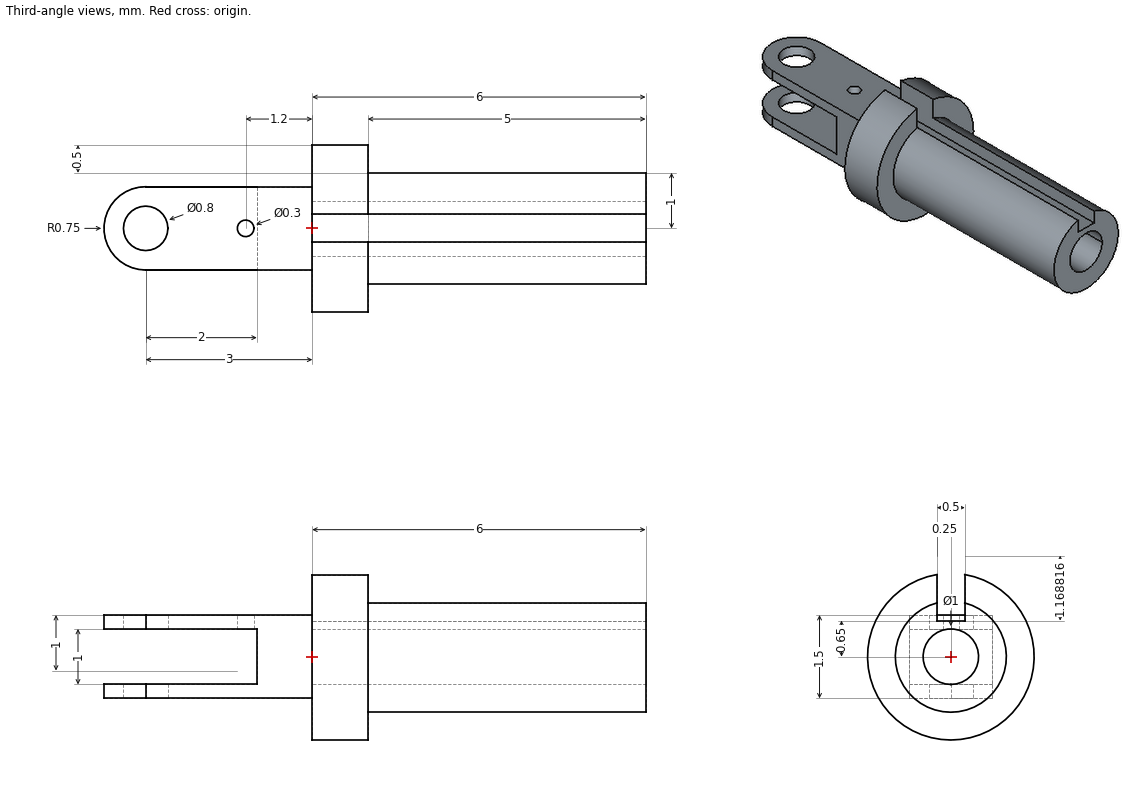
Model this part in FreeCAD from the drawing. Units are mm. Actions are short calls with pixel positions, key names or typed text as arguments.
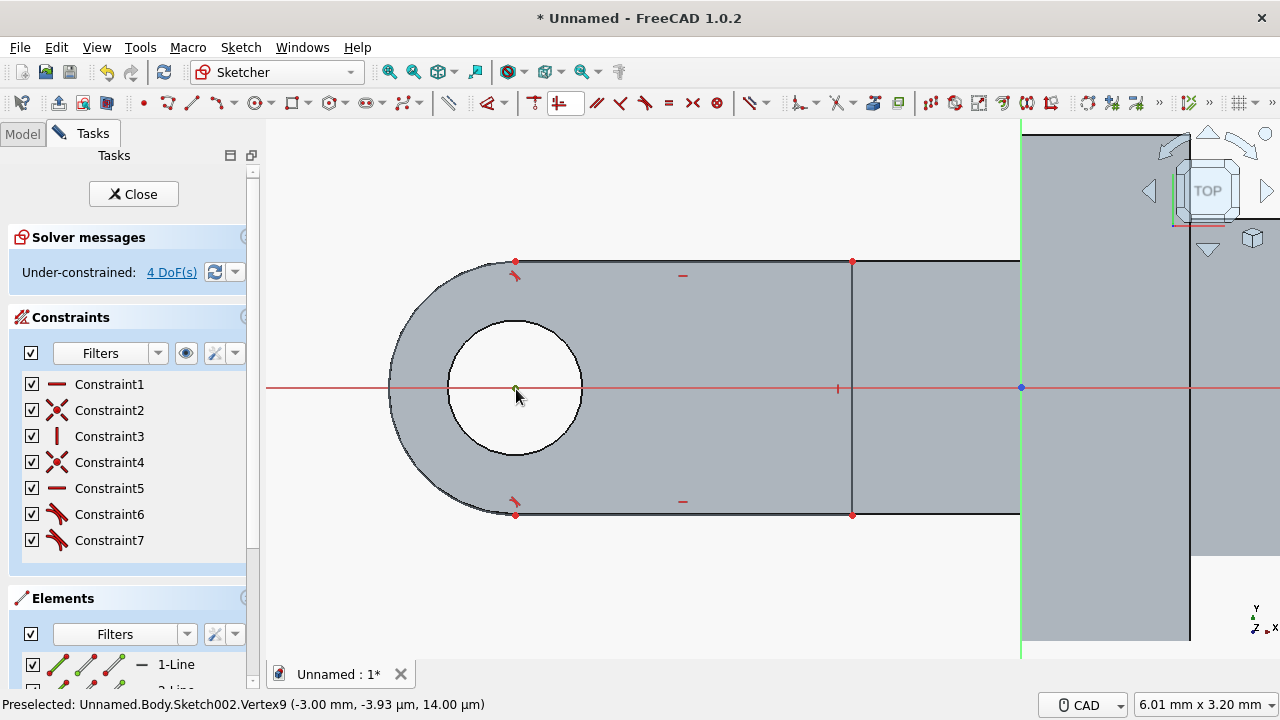
click(353, 388)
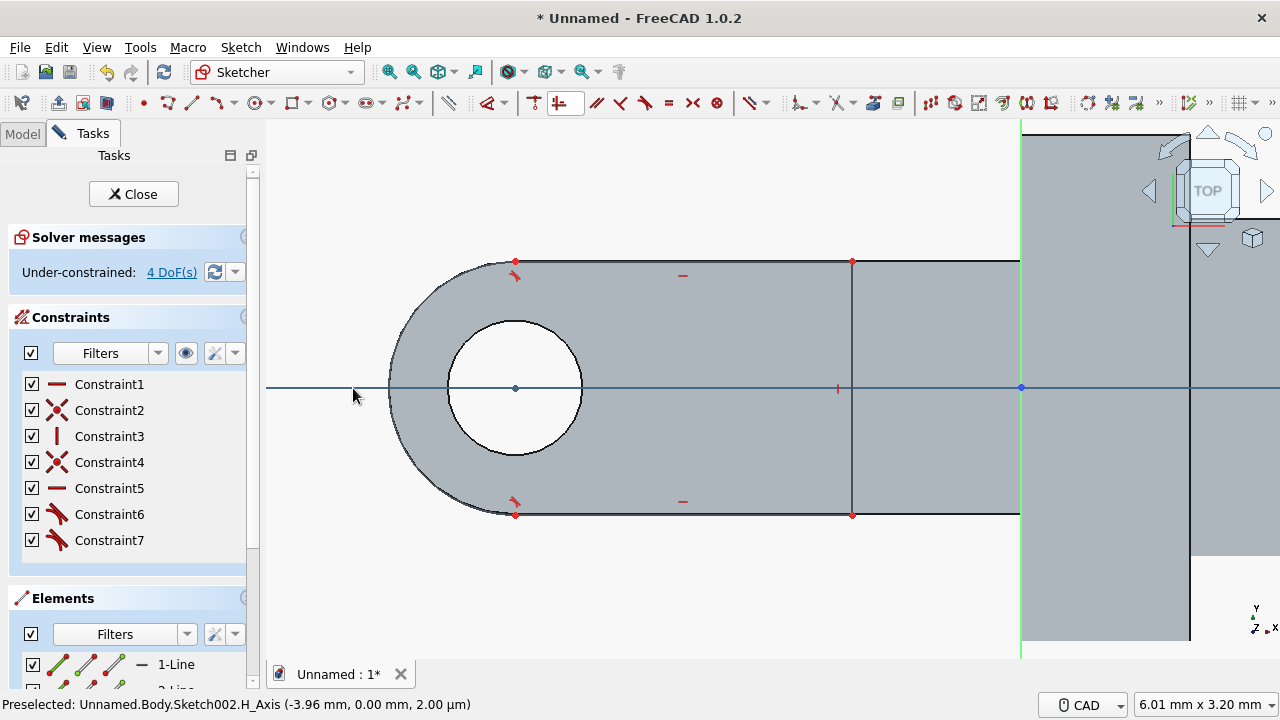
click(534, 104)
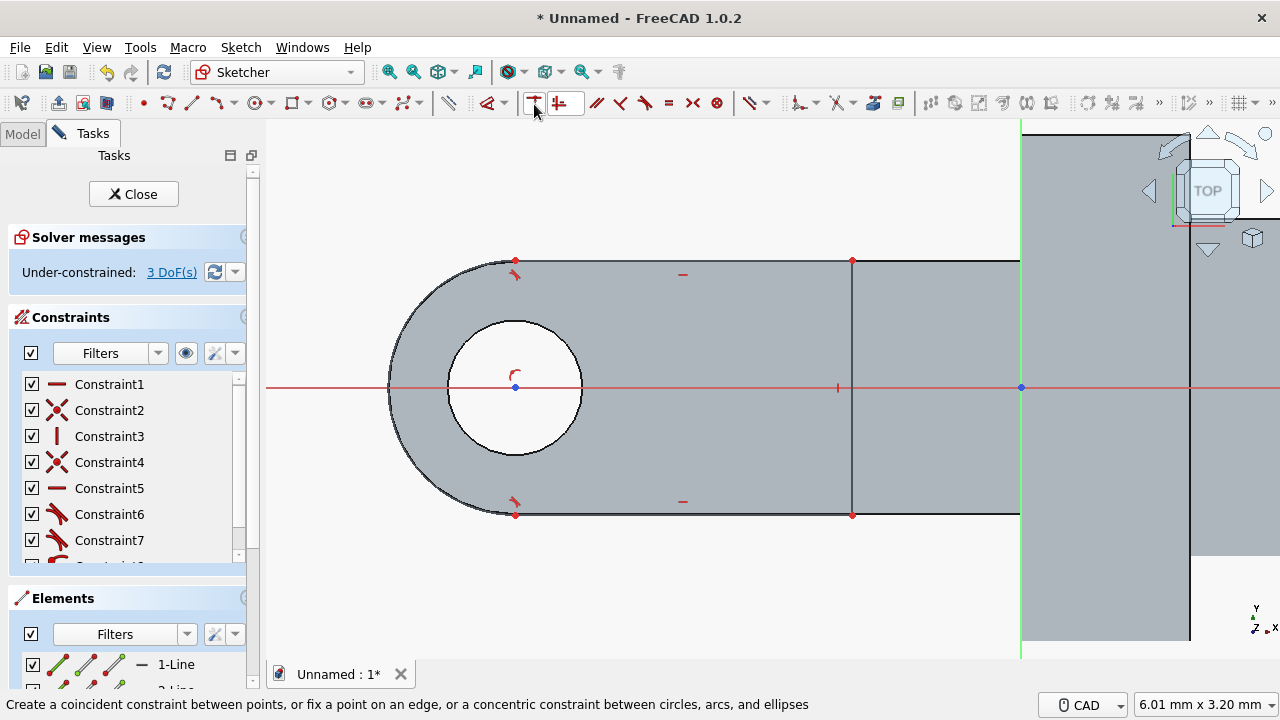
click(488, 104)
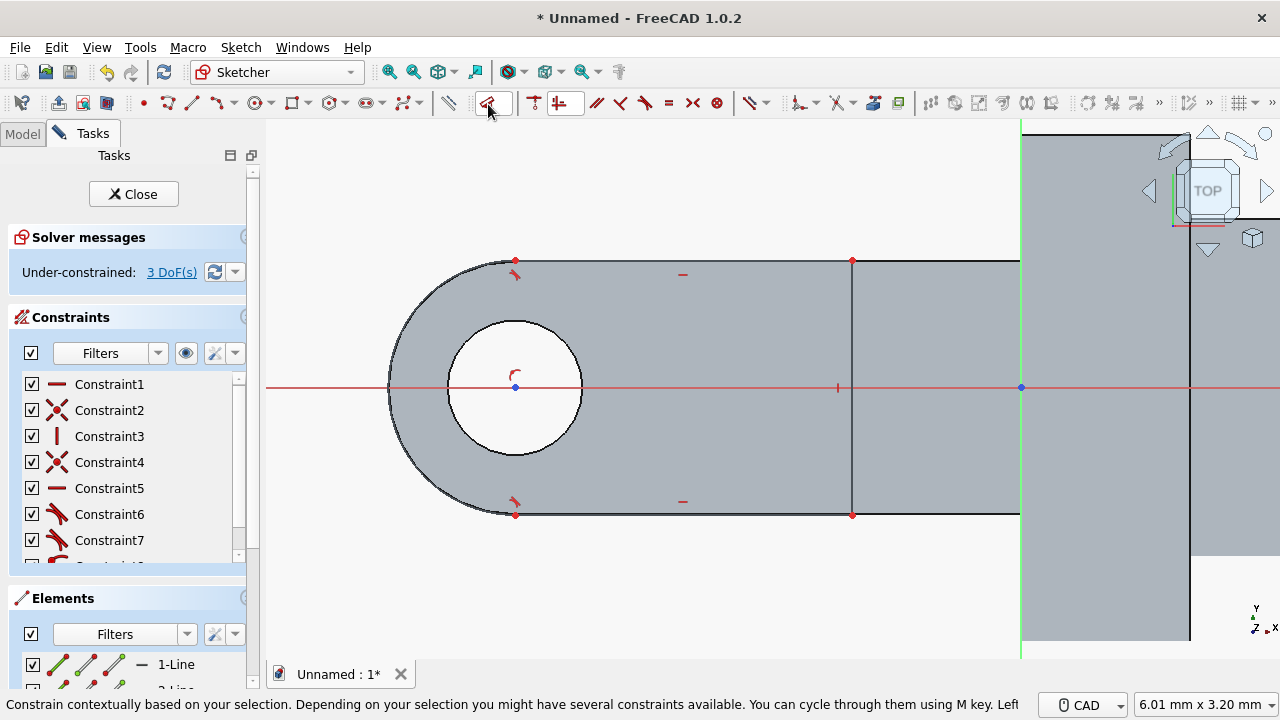
click(413, 313)
click(387, 294)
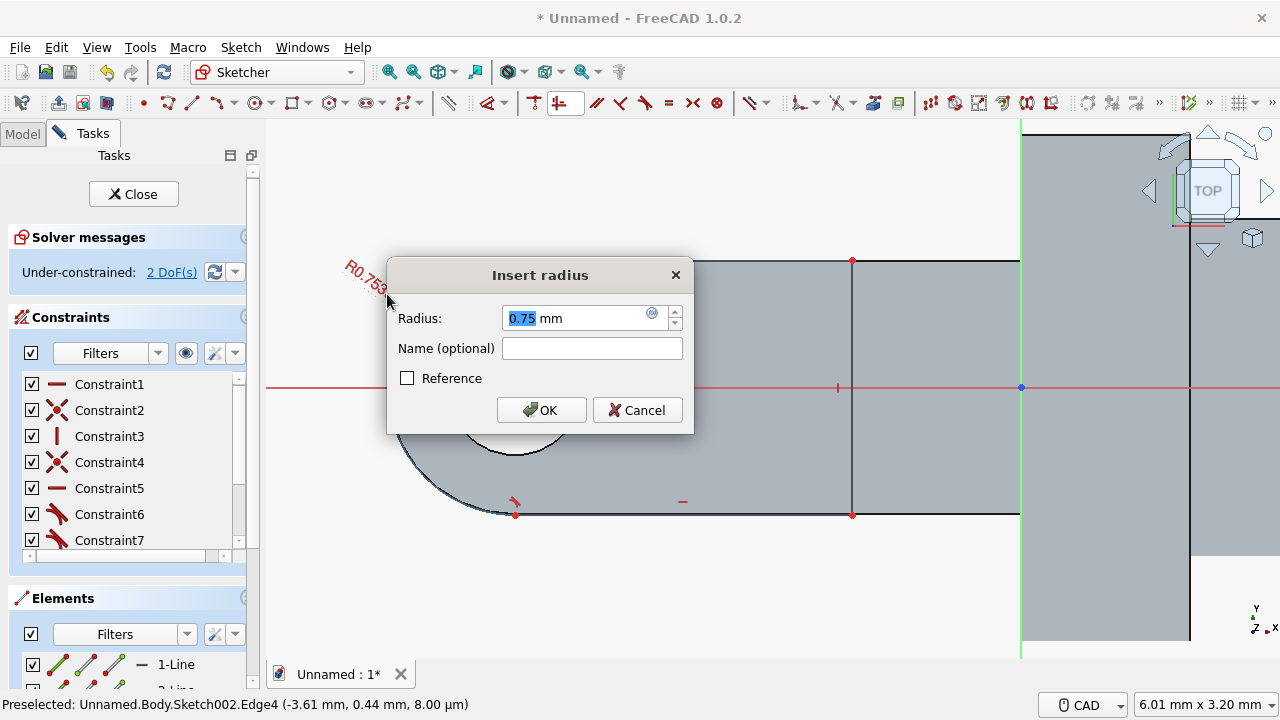
text(0.75)
key(Return)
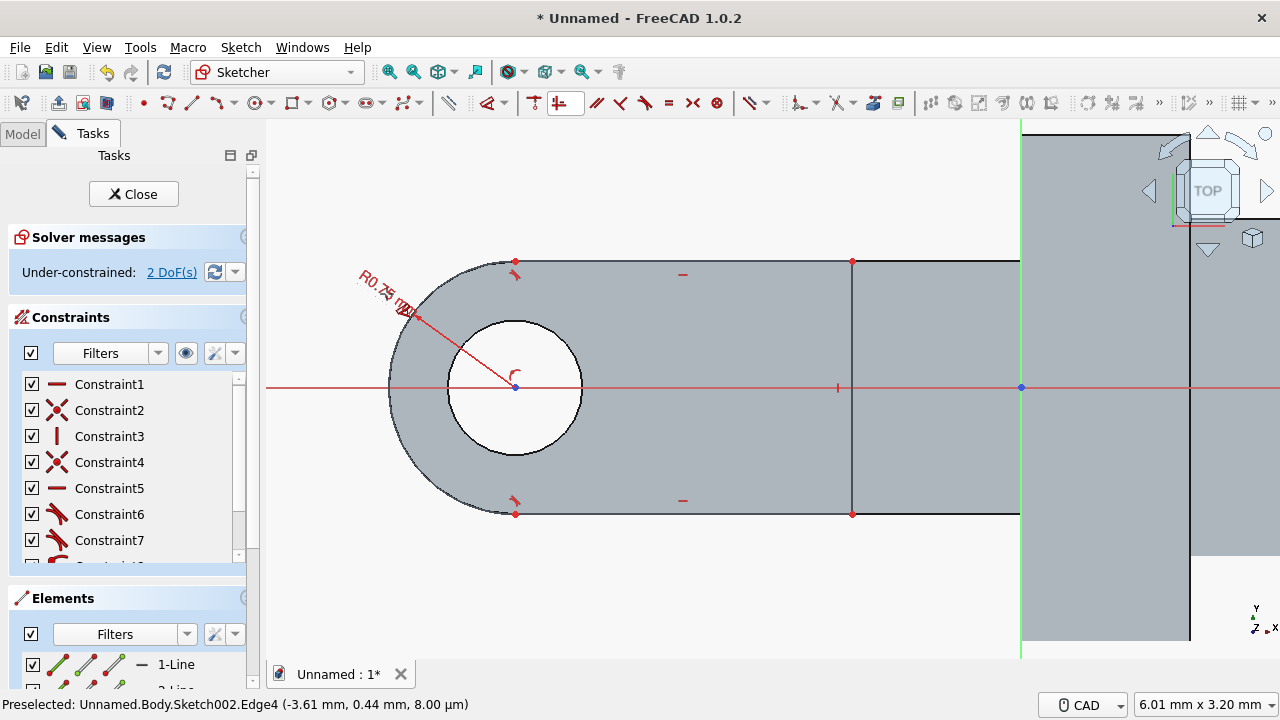
click(616, 514)
click(684, 548)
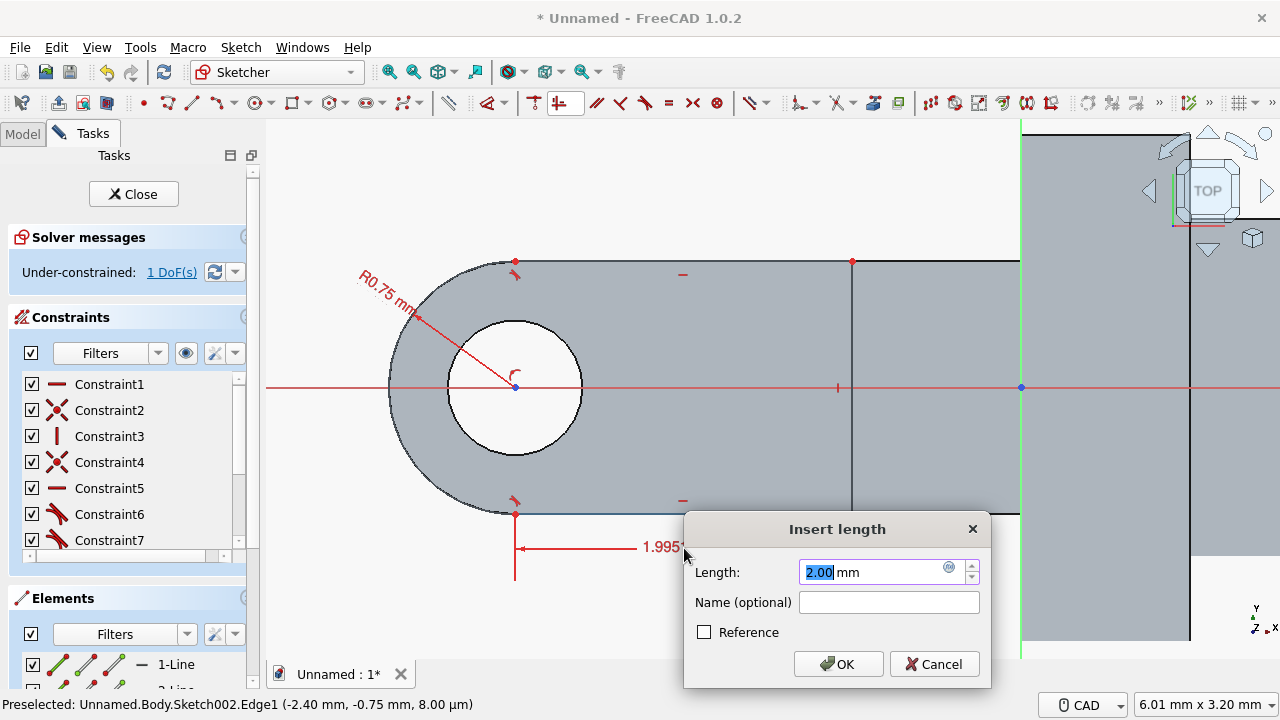
text(2)
key(Return)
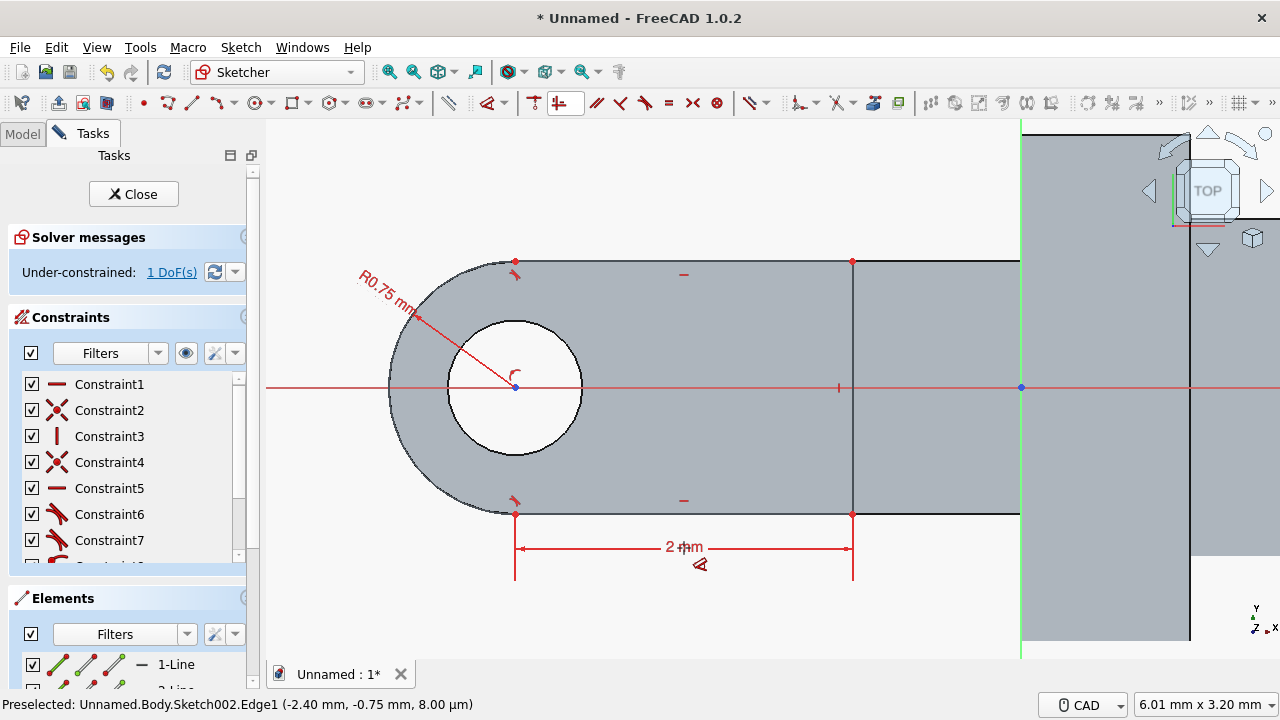
click(516, 514)
click(768, 548)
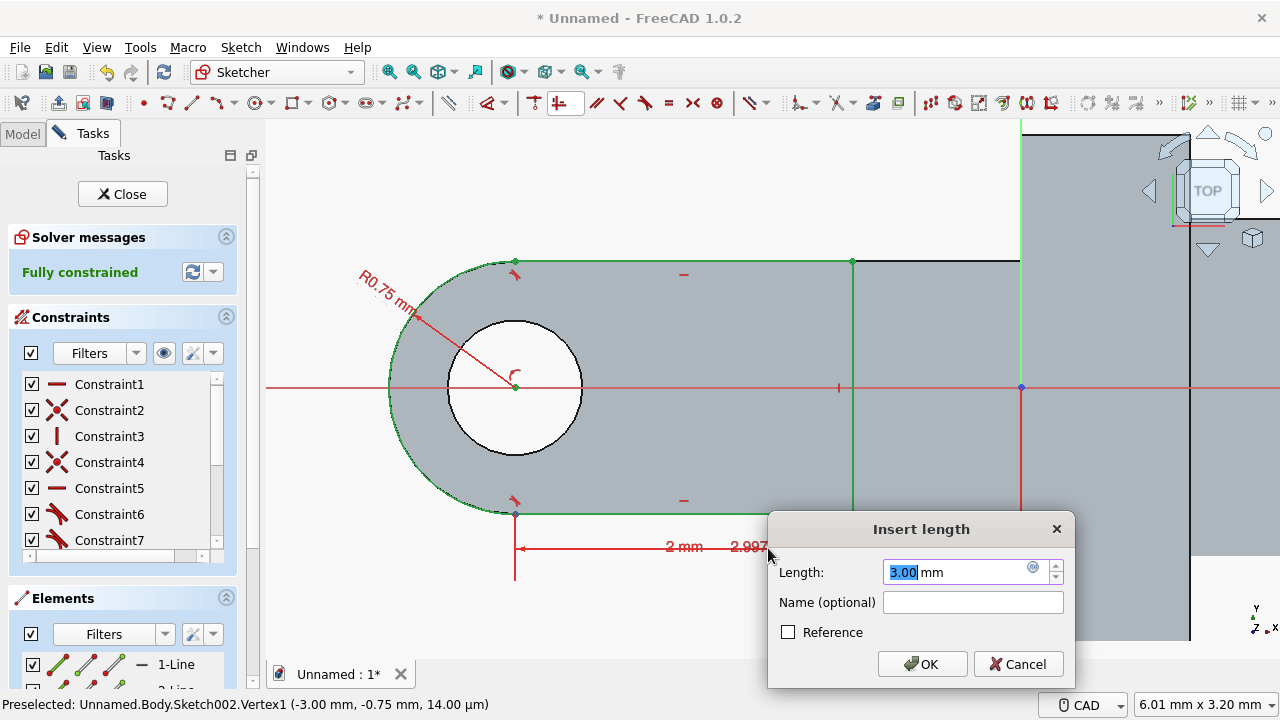
text(3)
key(Return)
key(Escape)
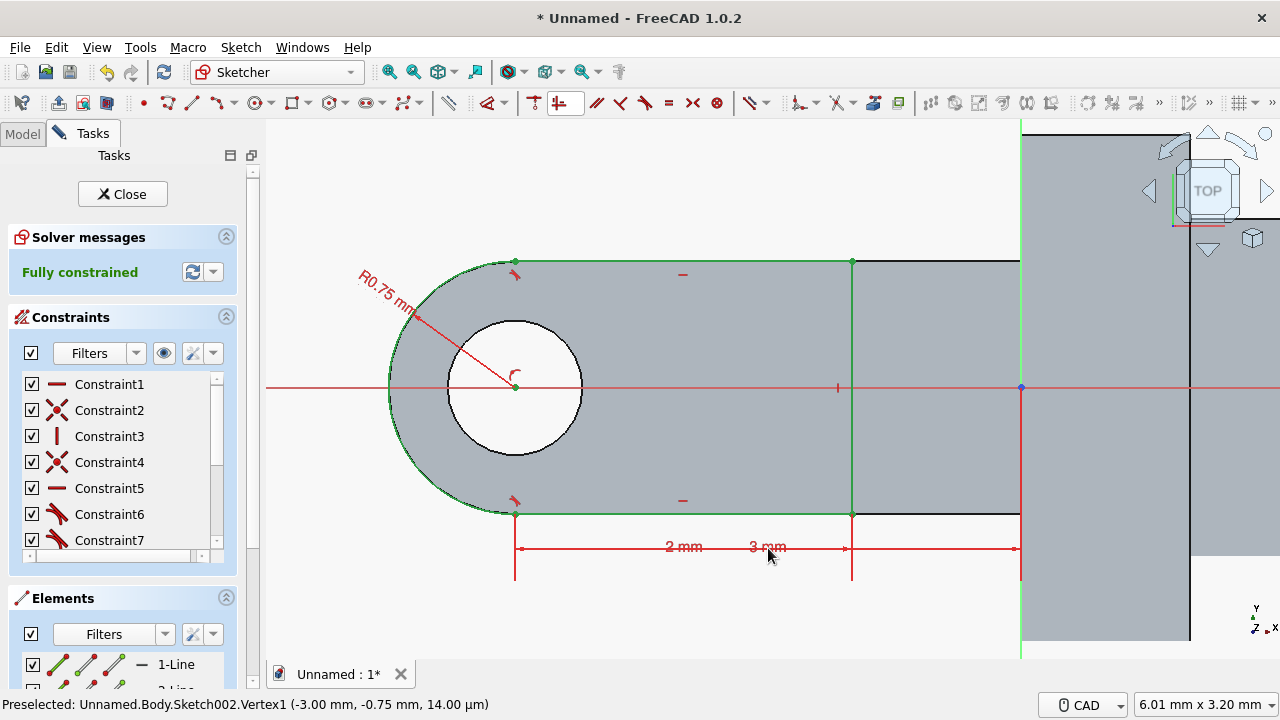
click(123, 194)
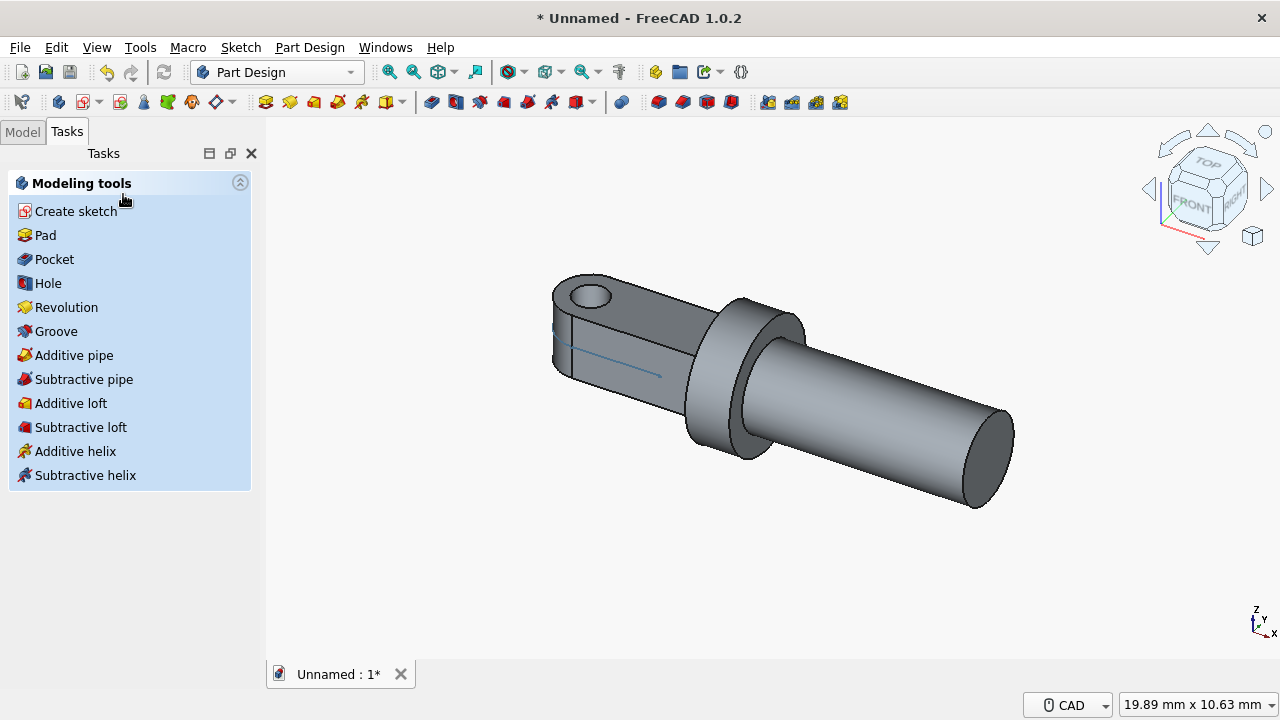
click(432, 102)